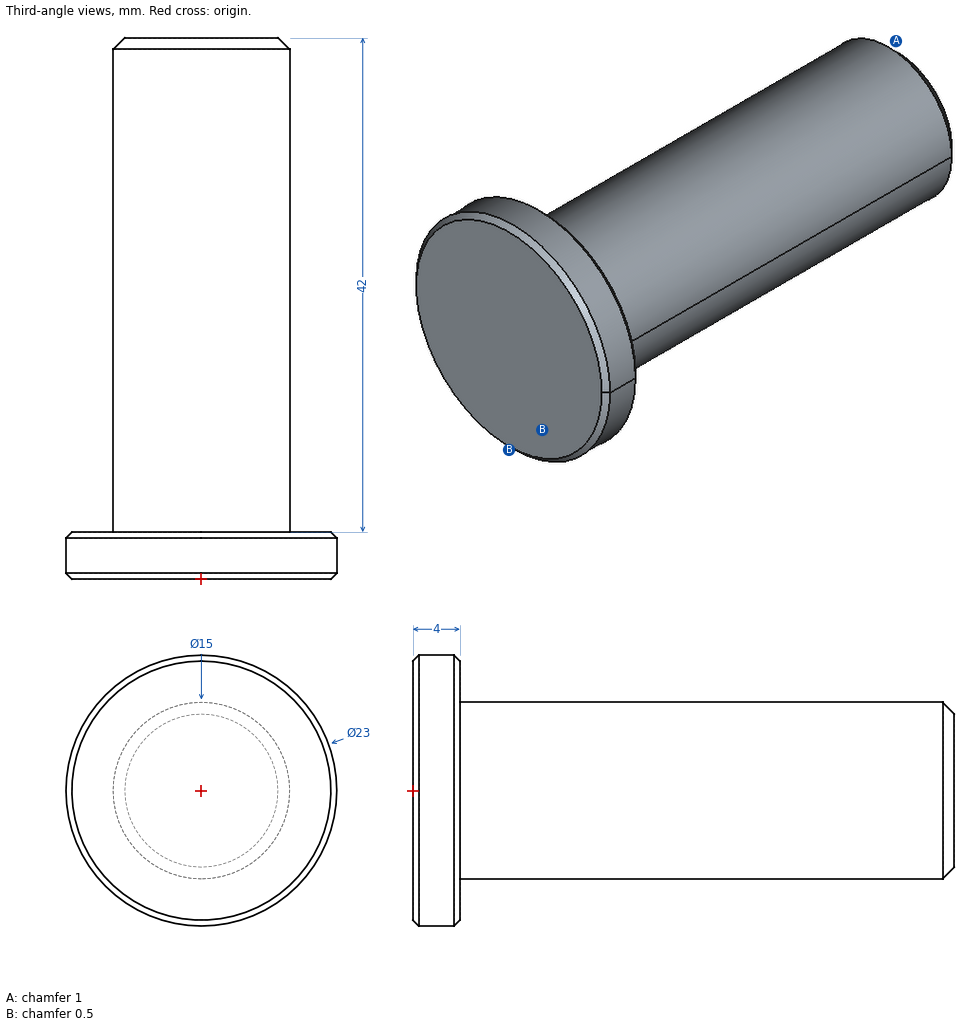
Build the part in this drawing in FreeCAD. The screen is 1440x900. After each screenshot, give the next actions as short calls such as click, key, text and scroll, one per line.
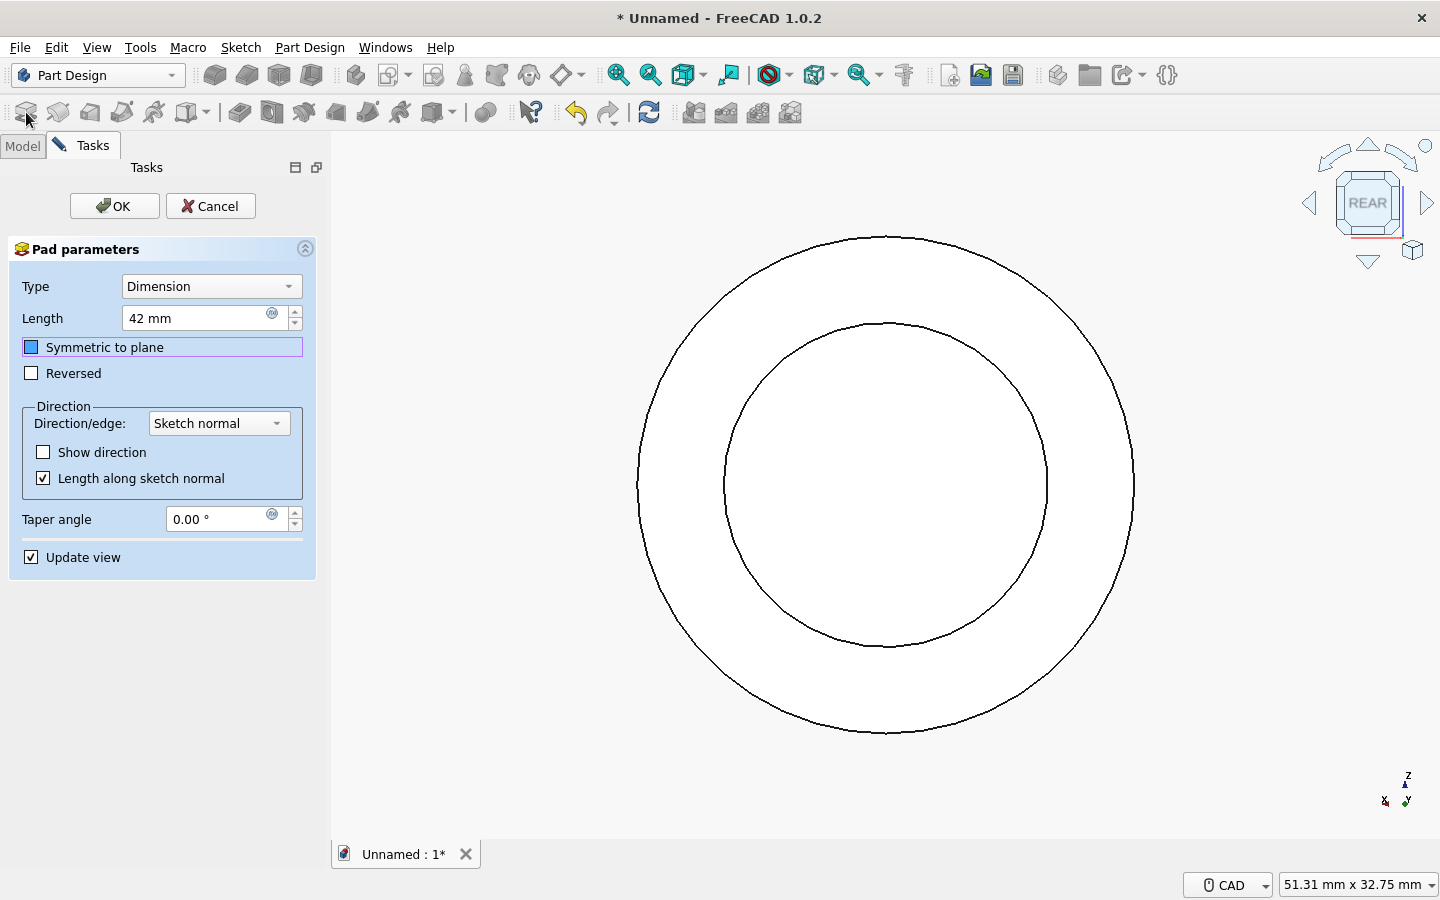
click(115, 206)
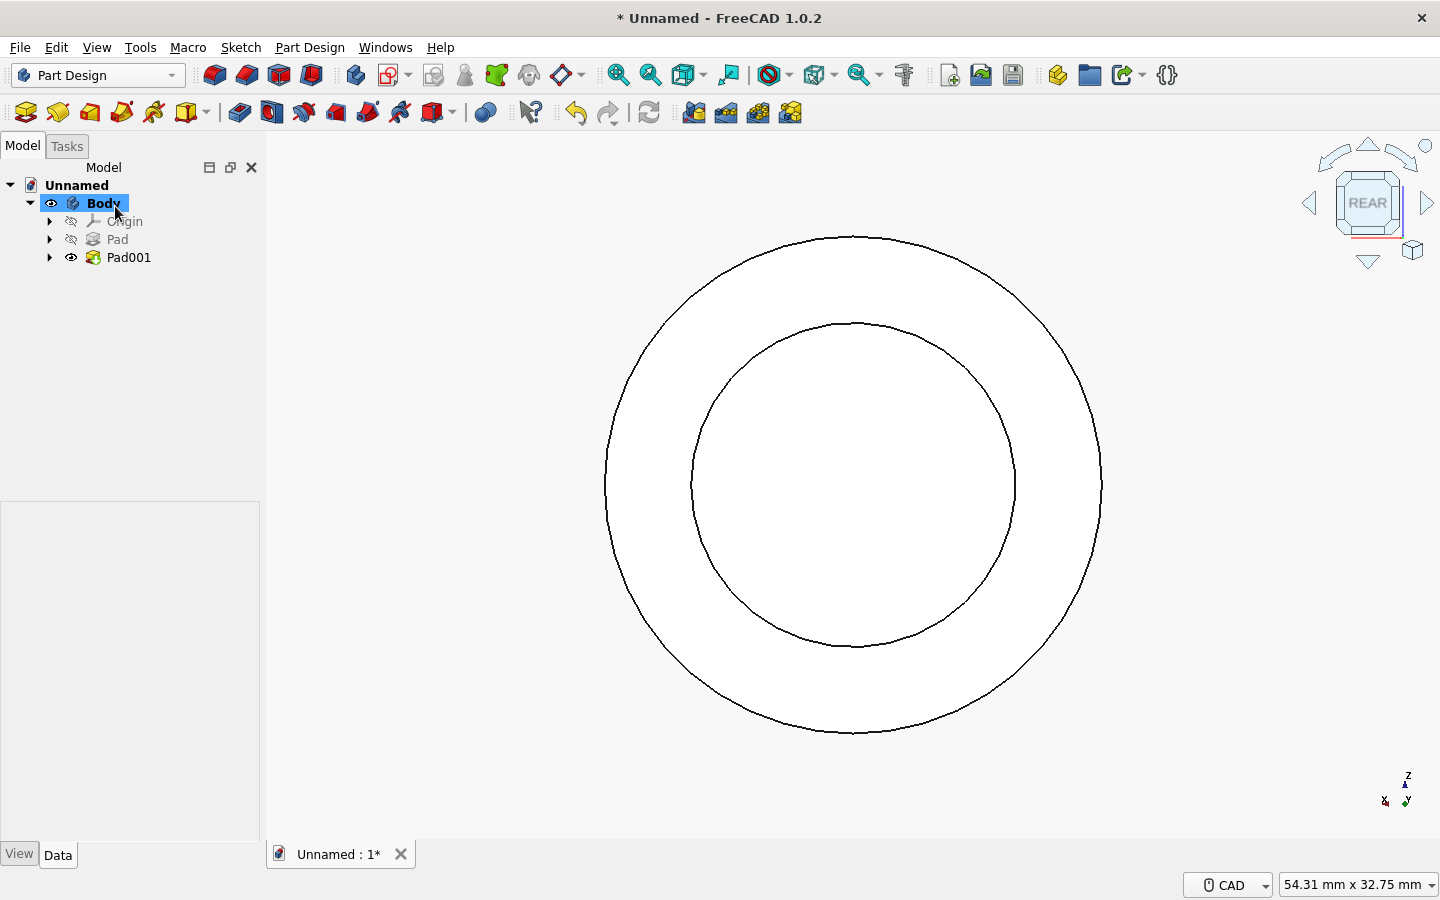
click(1015, 484)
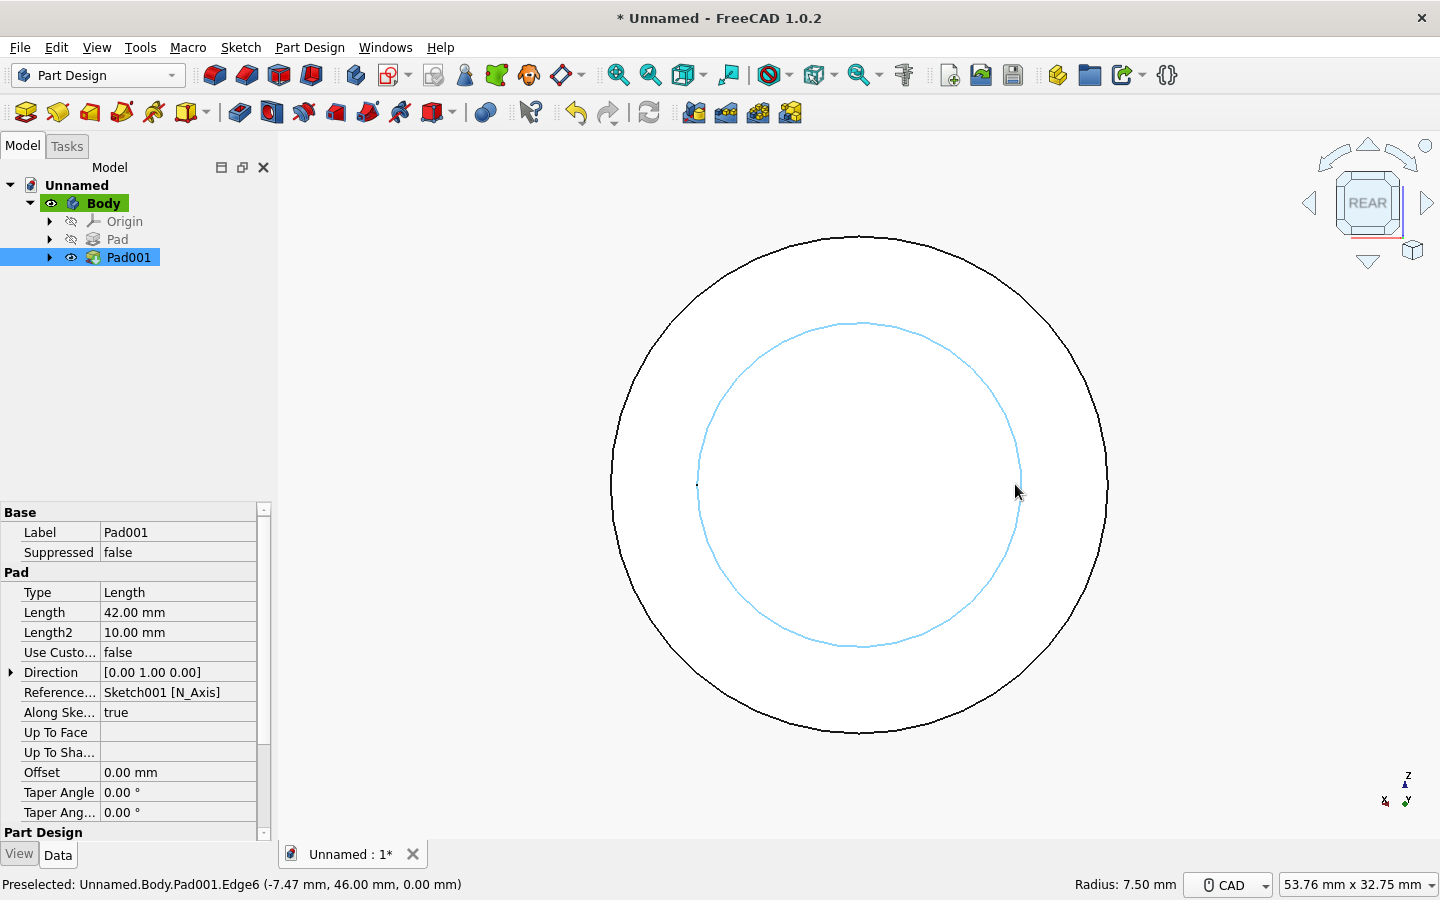
click(248, 76)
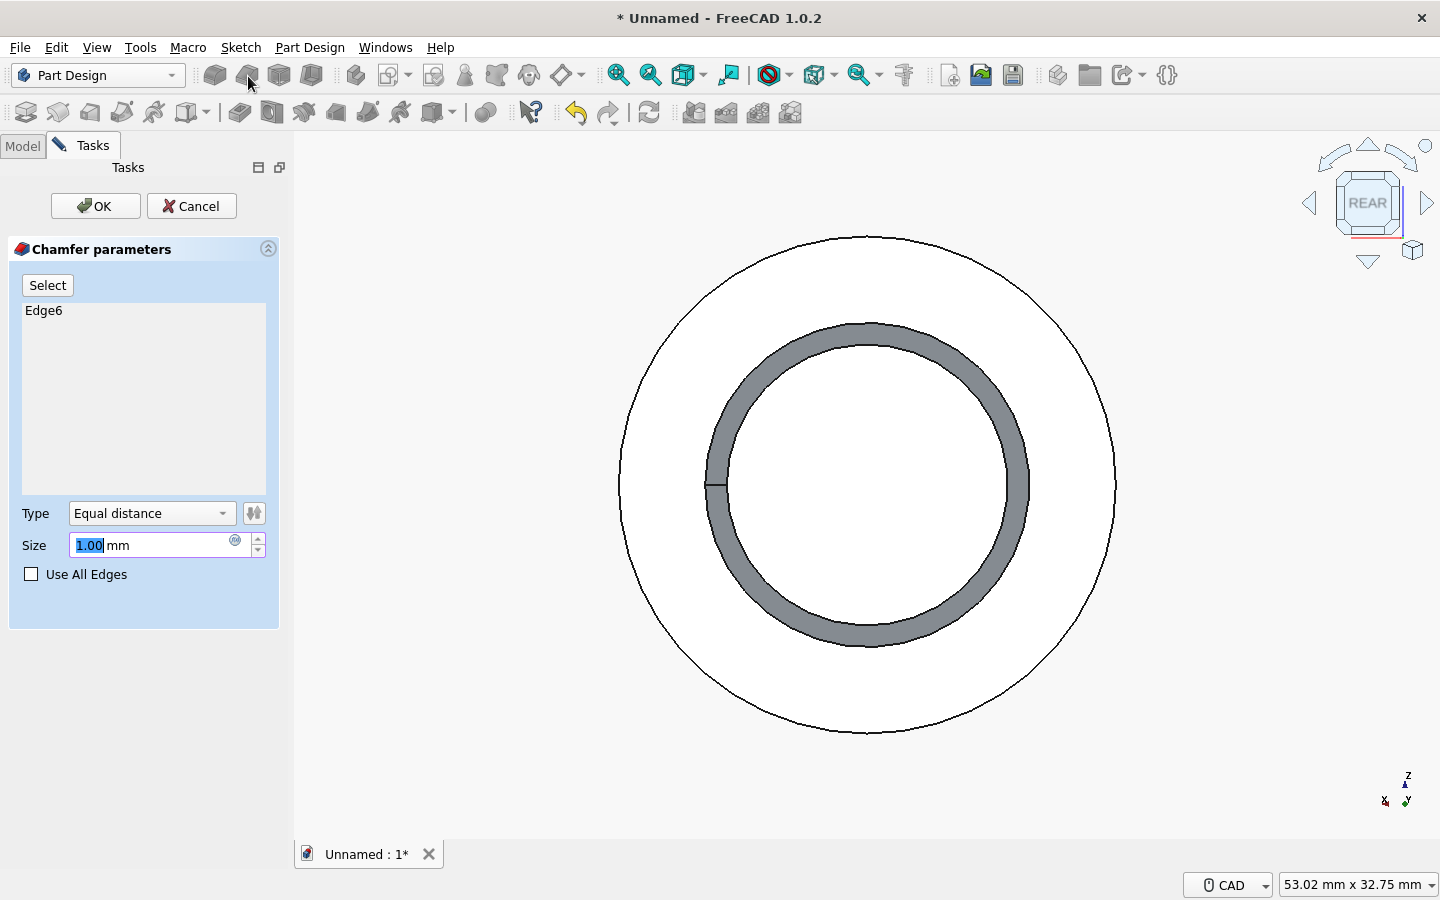
text(1)
key(Tab)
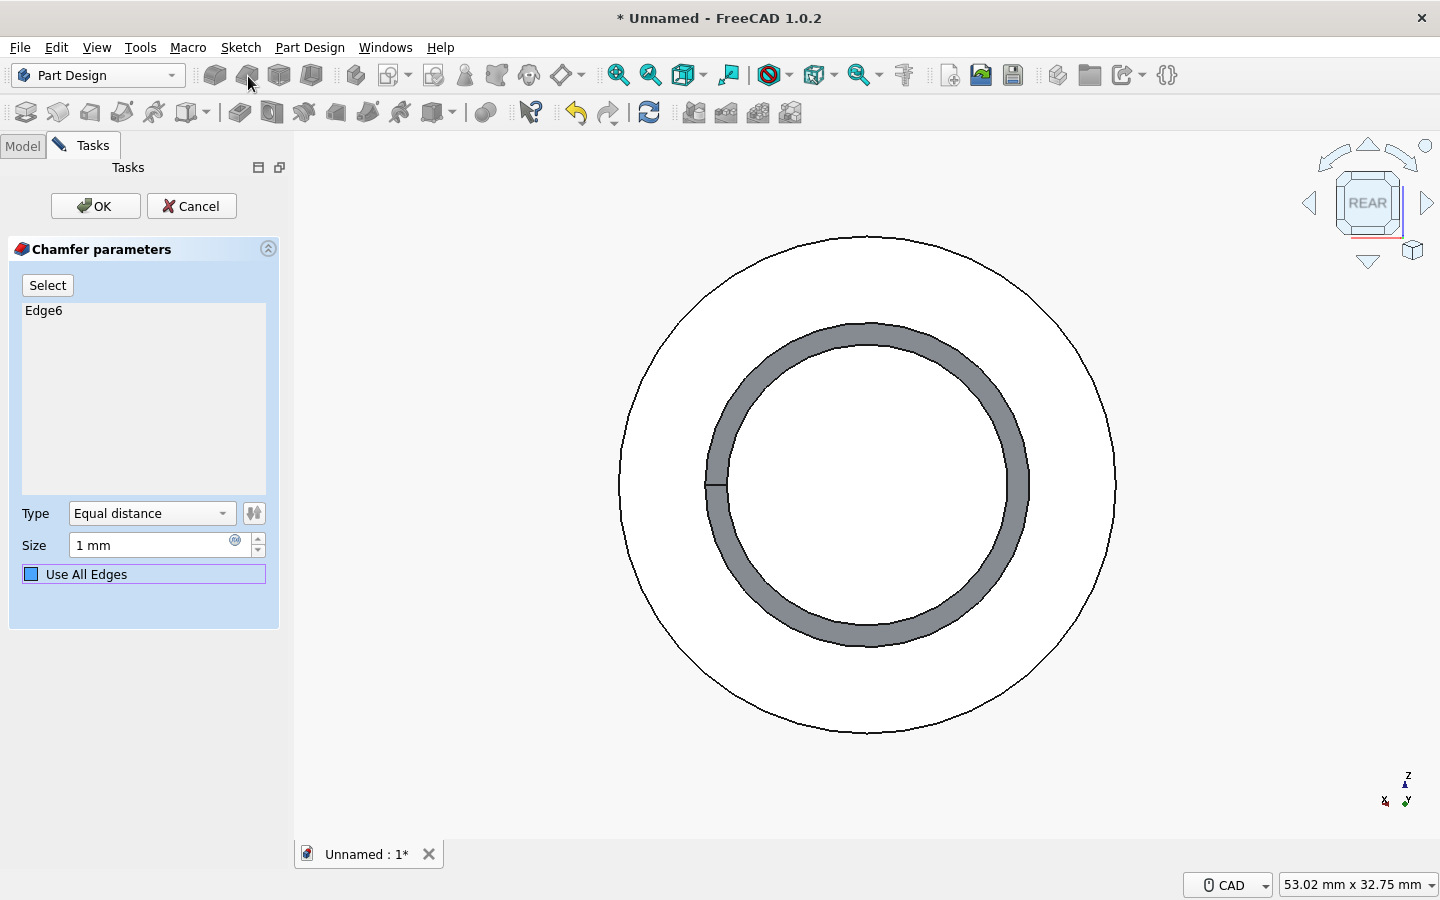
click(96, 206)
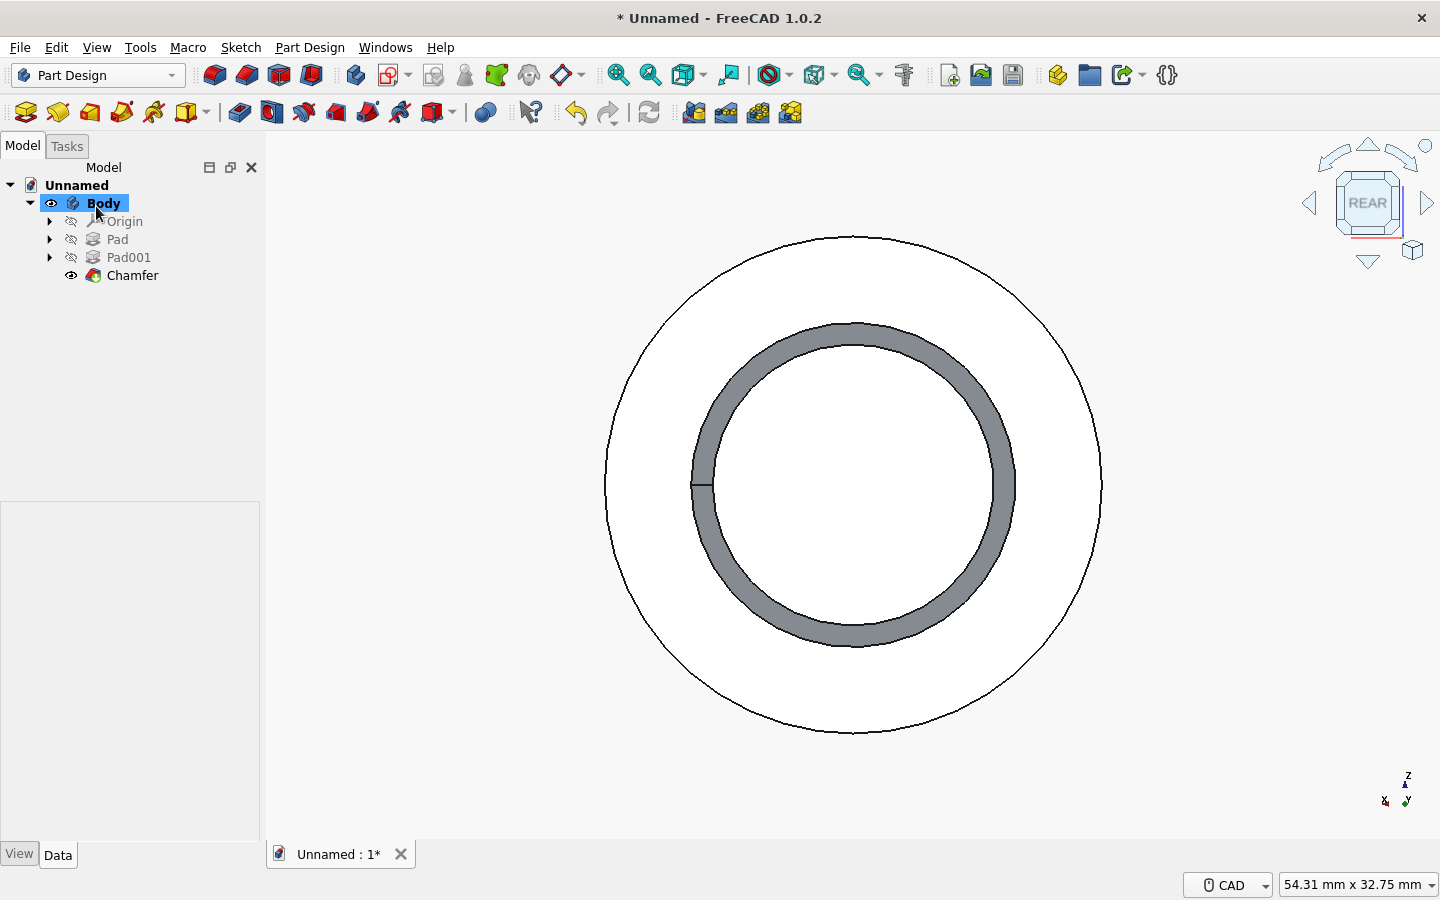
click(1102, 484)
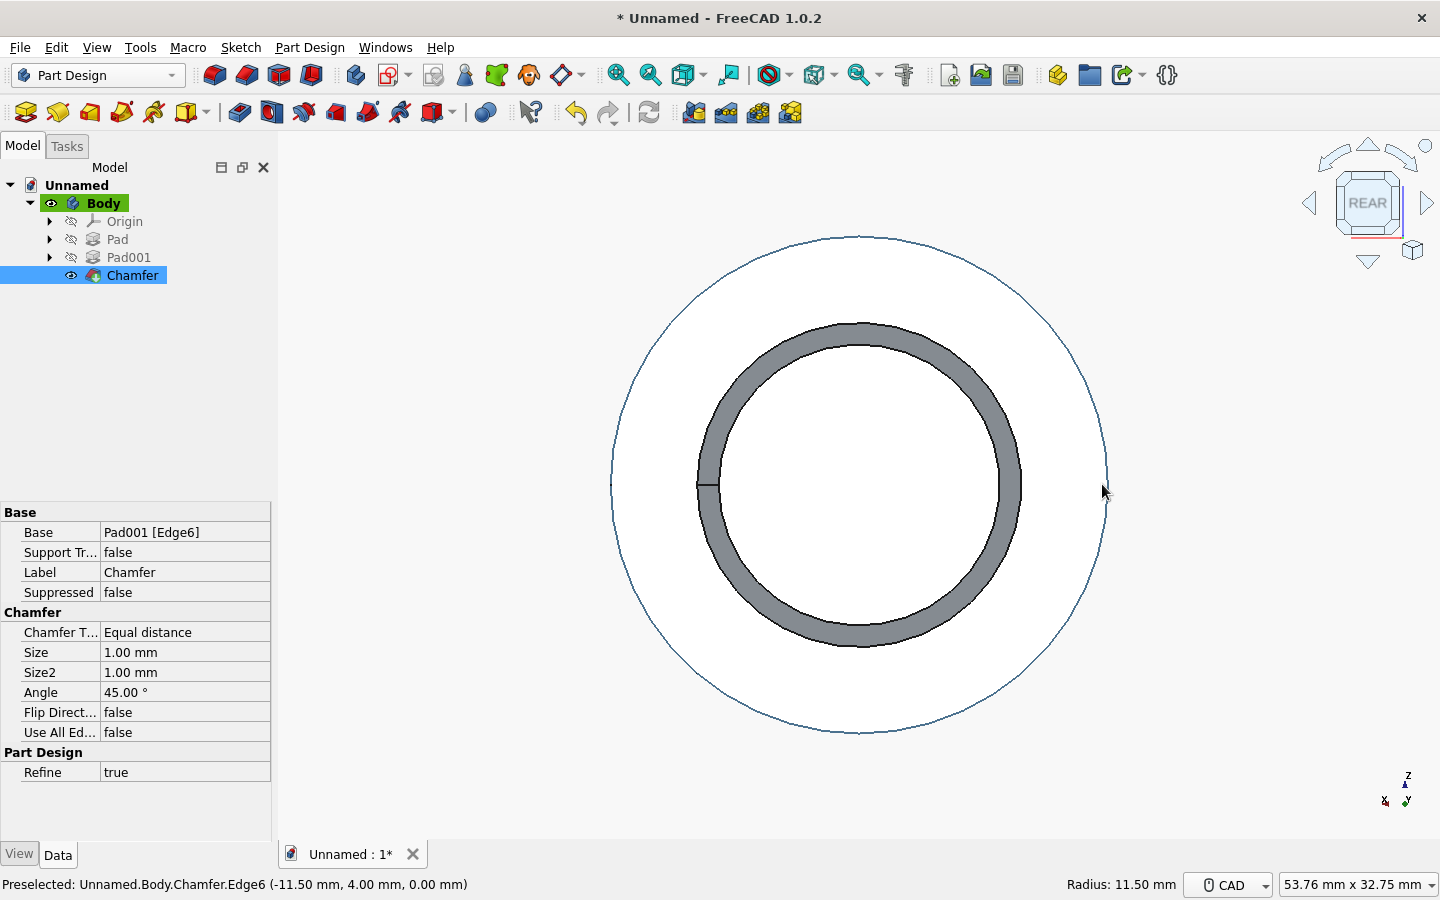
key(0)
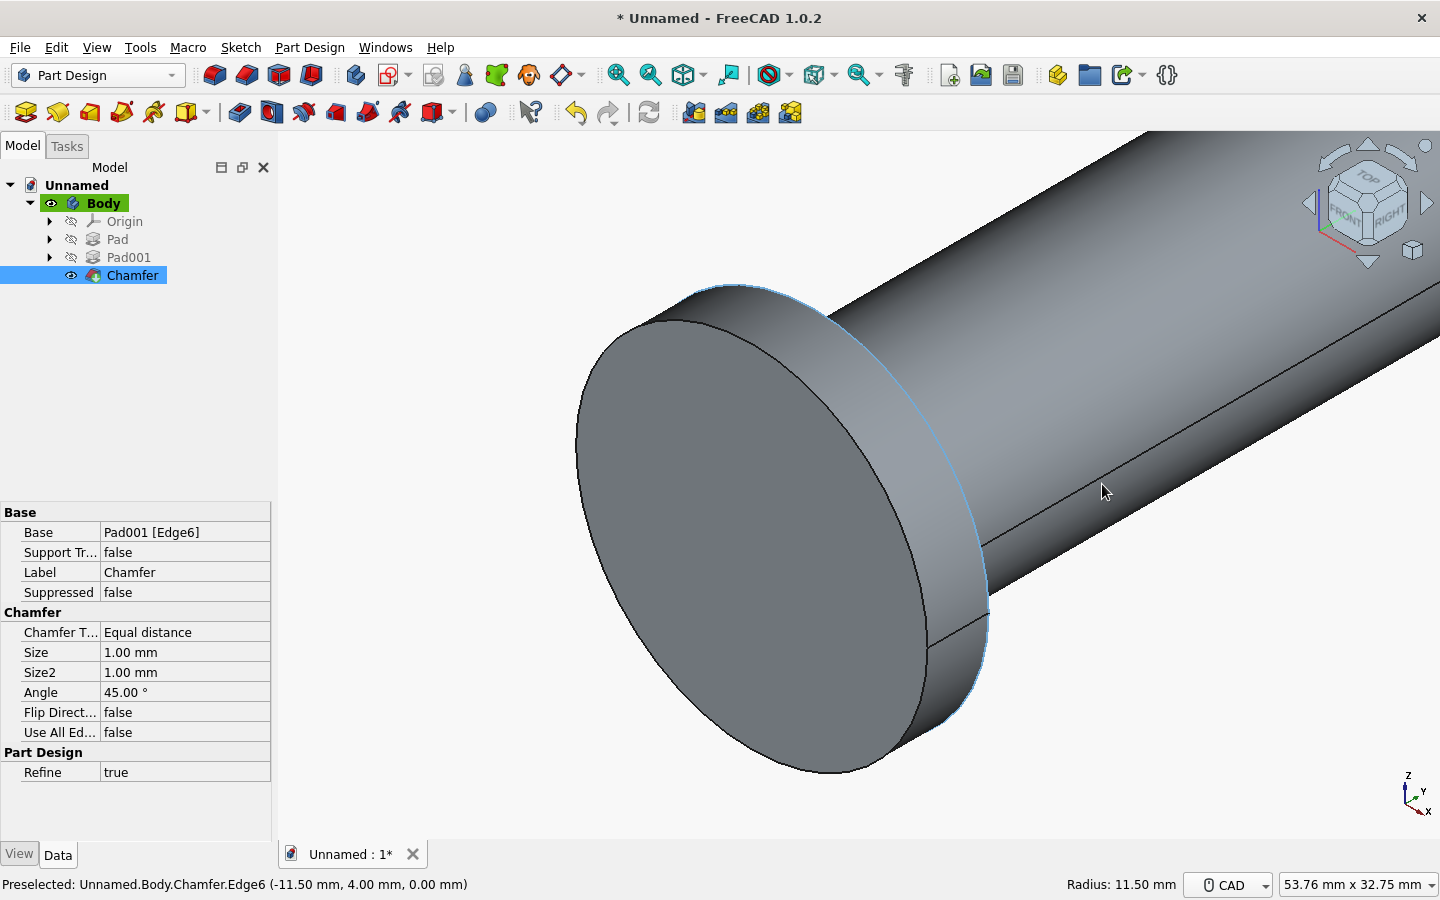
click(620, 76)